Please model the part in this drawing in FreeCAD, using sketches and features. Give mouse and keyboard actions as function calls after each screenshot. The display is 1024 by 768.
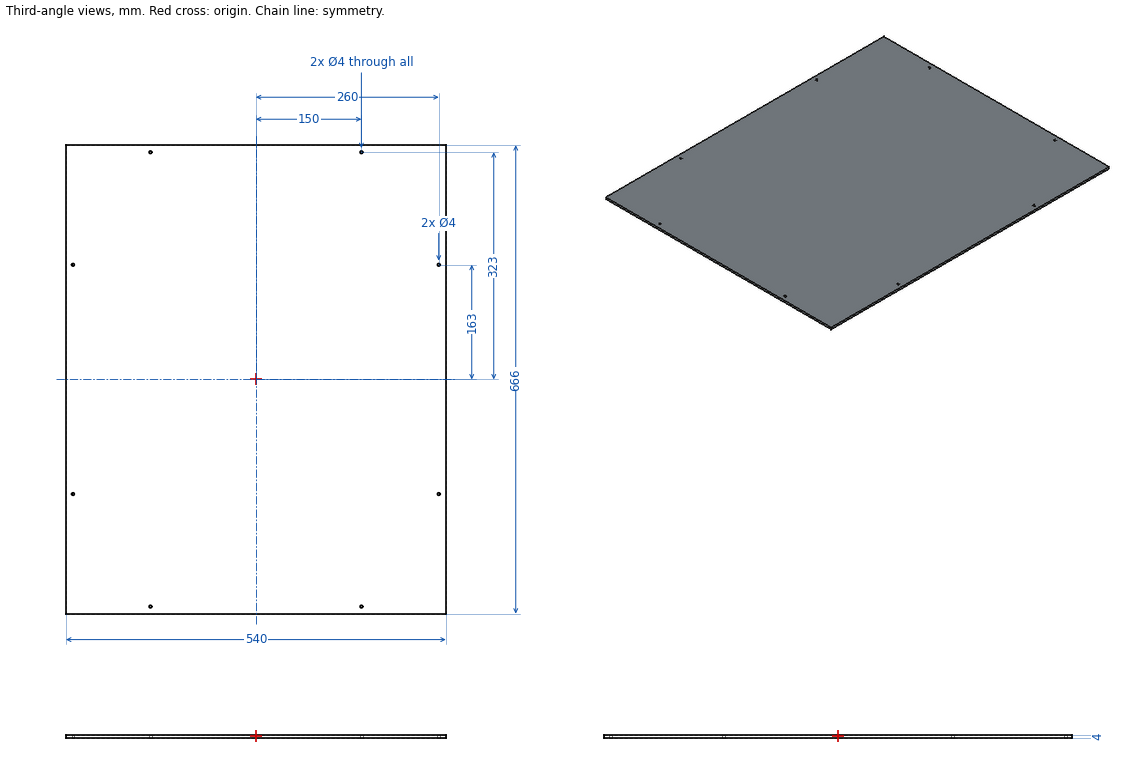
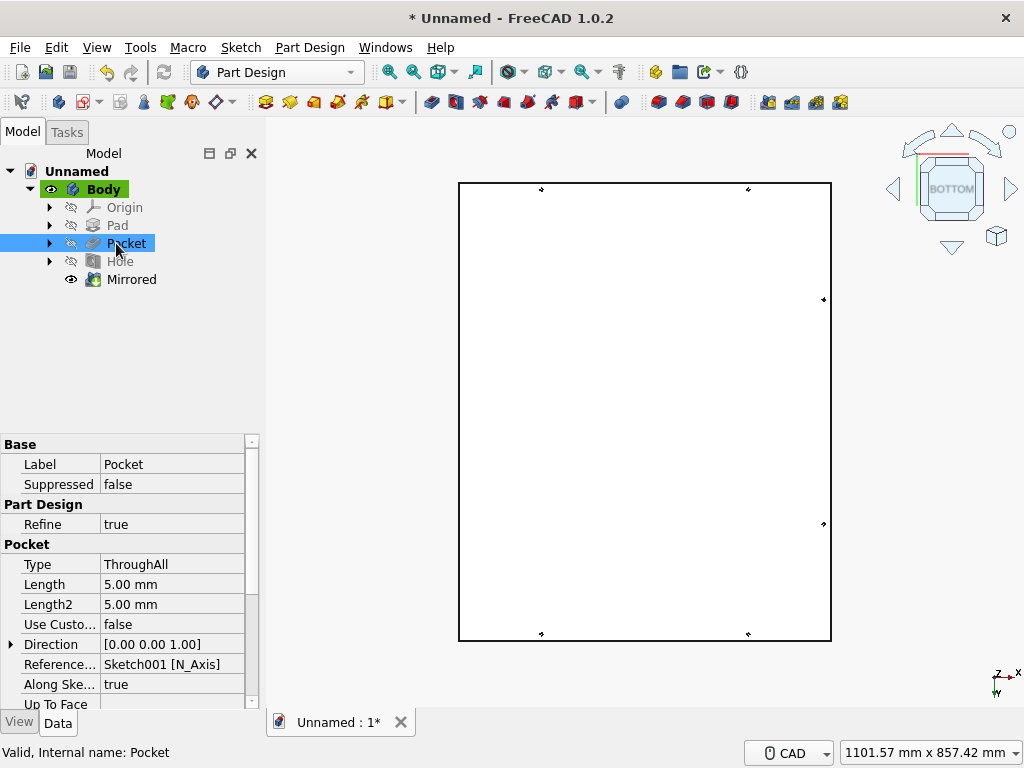
click(768, 102)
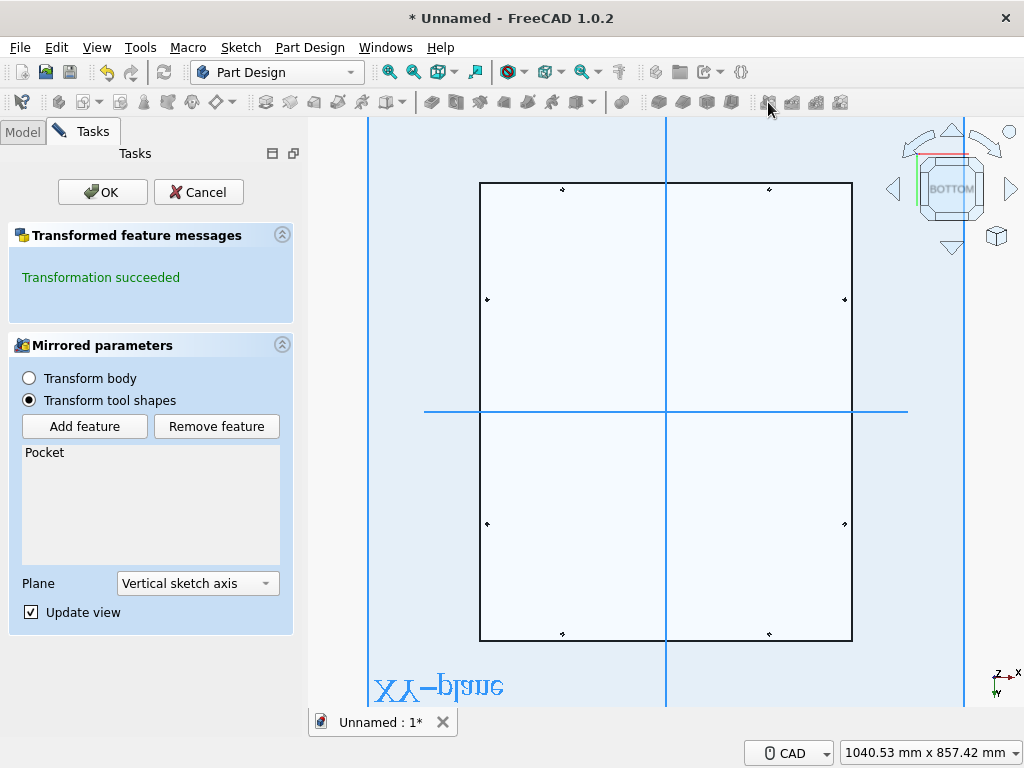
click(198, 584)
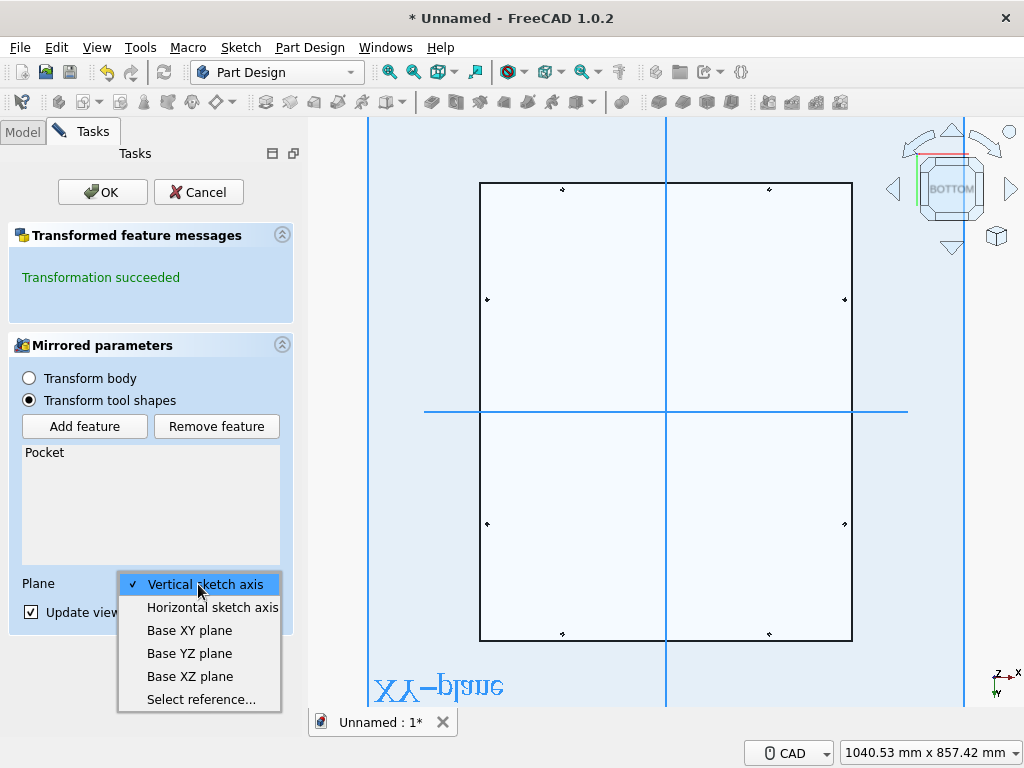
click(198, 654)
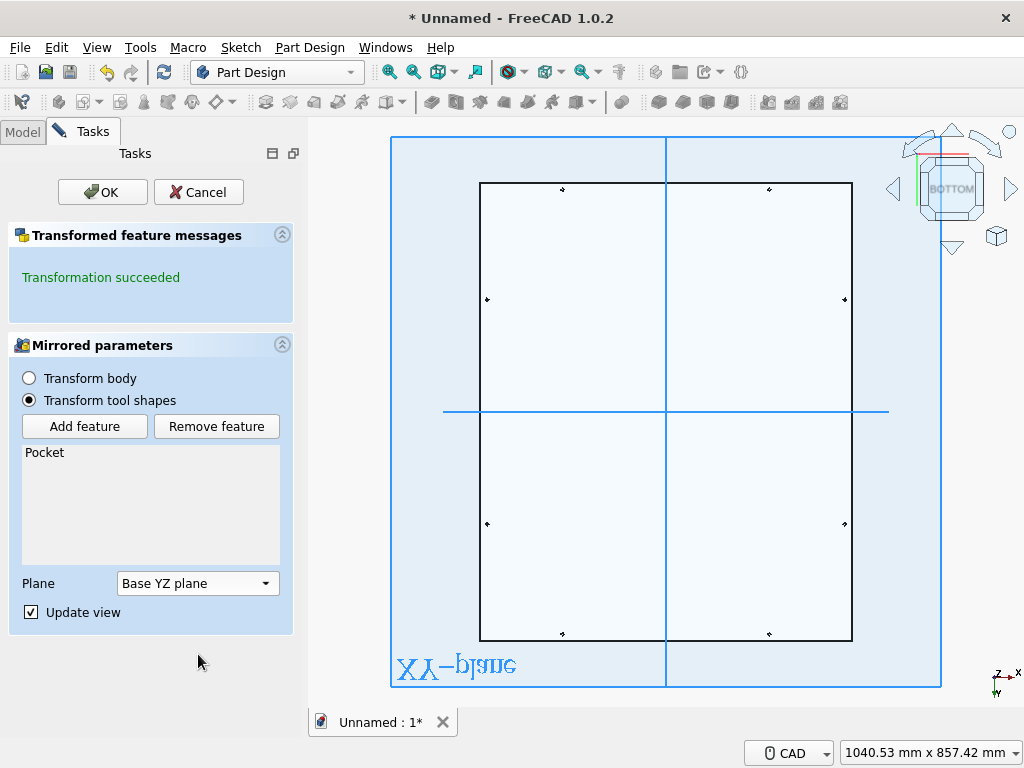
click(103, 192)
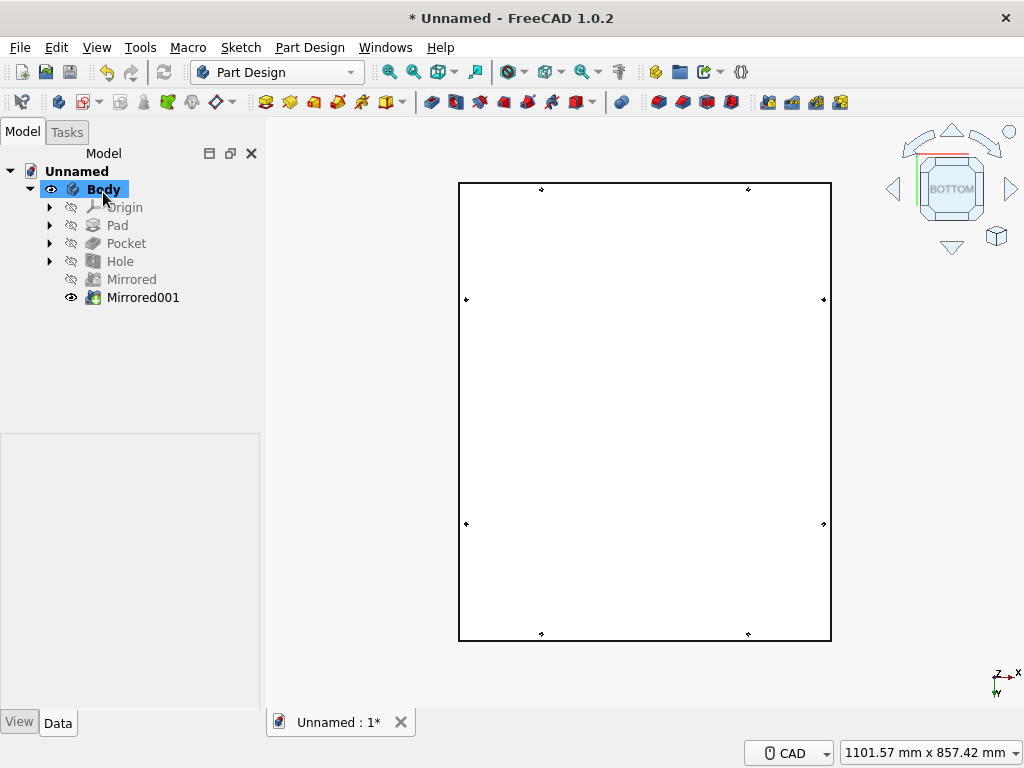
key(0)